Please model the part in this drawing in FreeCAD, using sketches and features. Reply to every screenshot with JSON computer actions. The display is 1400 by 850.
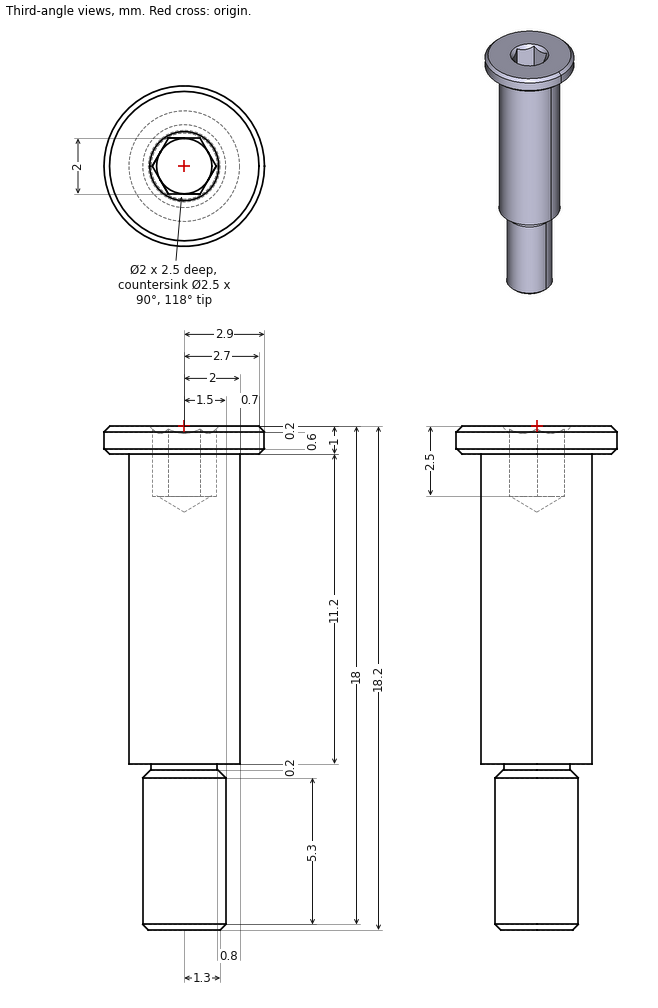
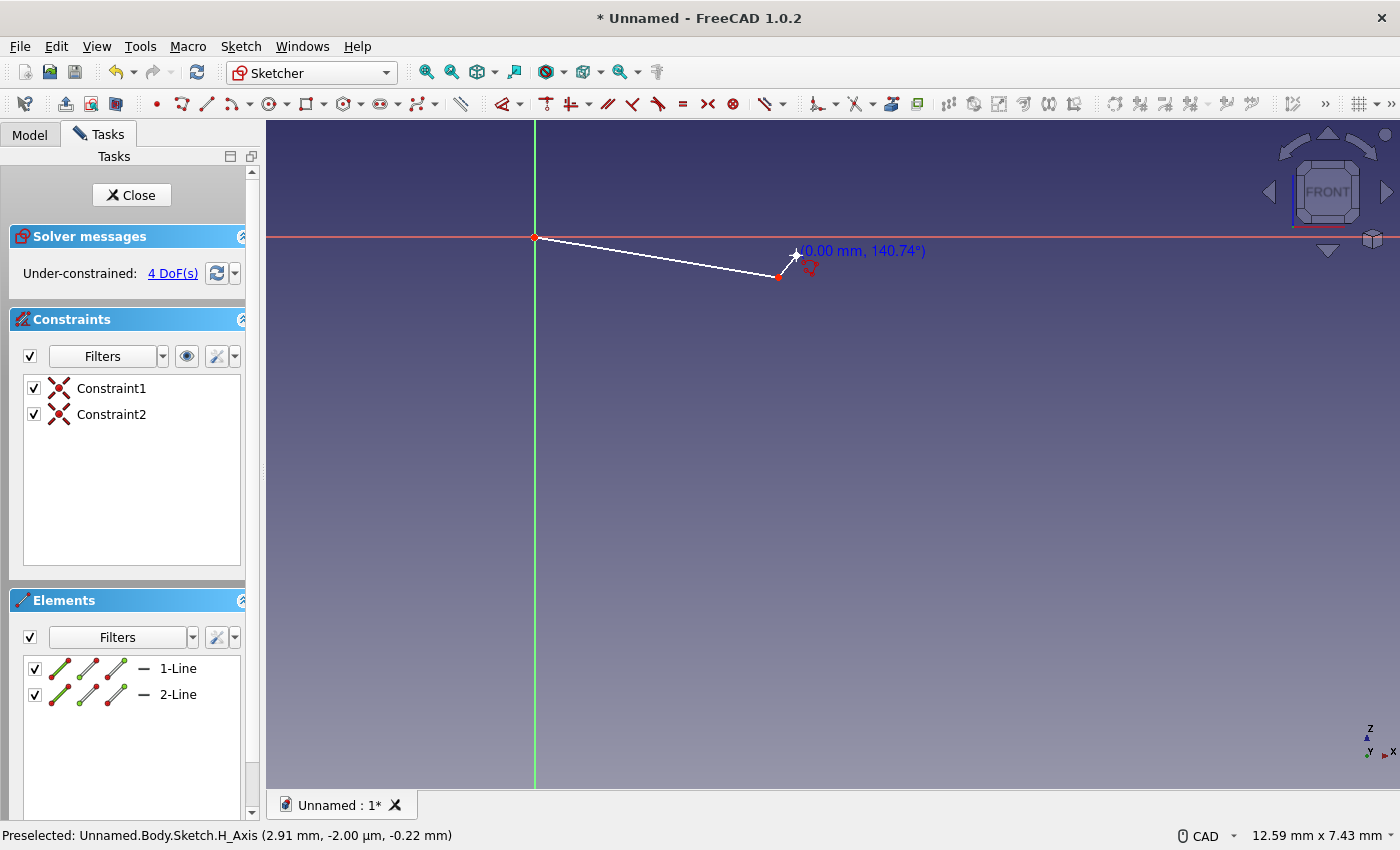
{"action": "scroll", "coordinate": [797, 257], "scroll_direction": "down", "scroll_amount": 7}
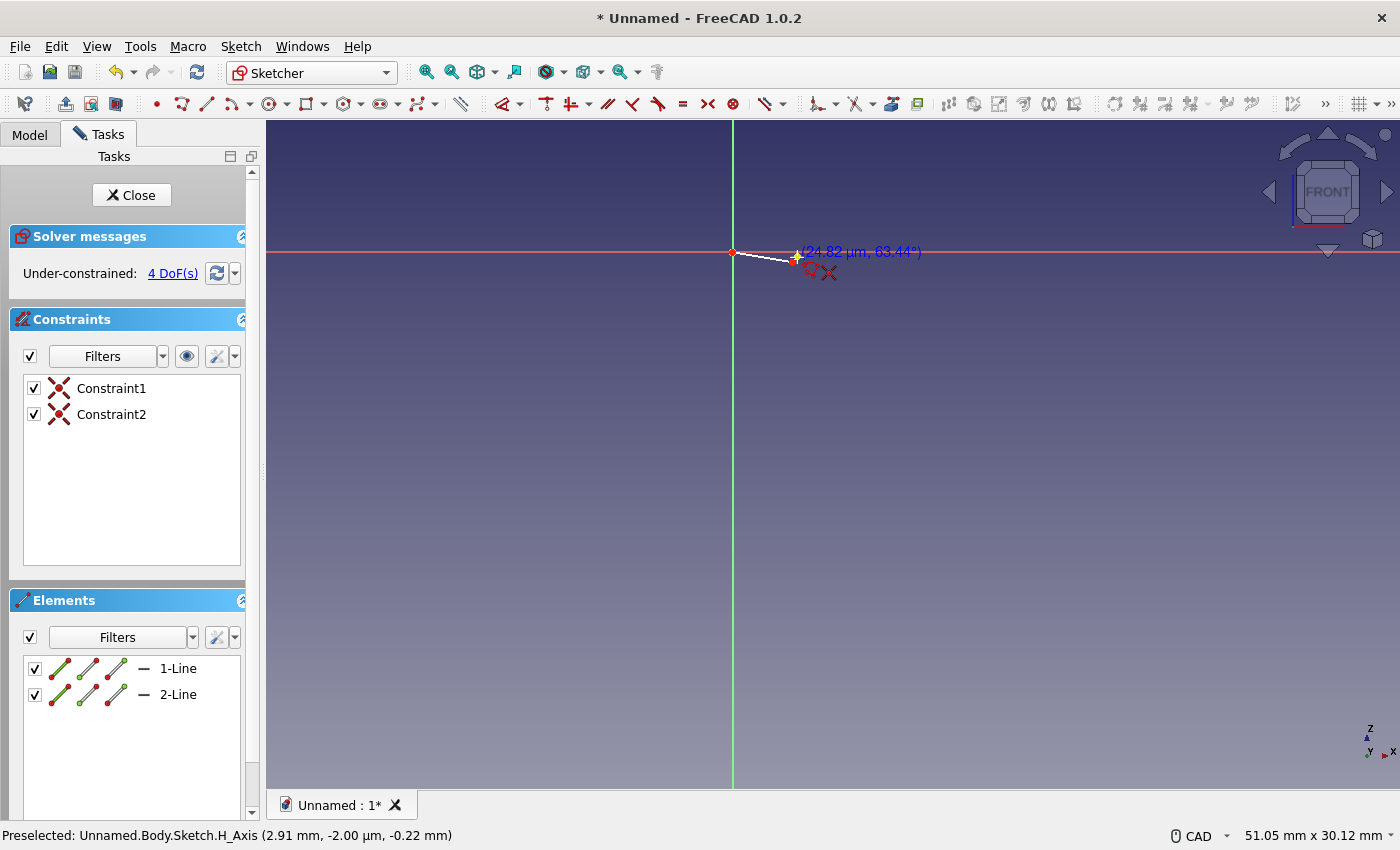
{"action": "left_click", "coordinate": [797, 270]}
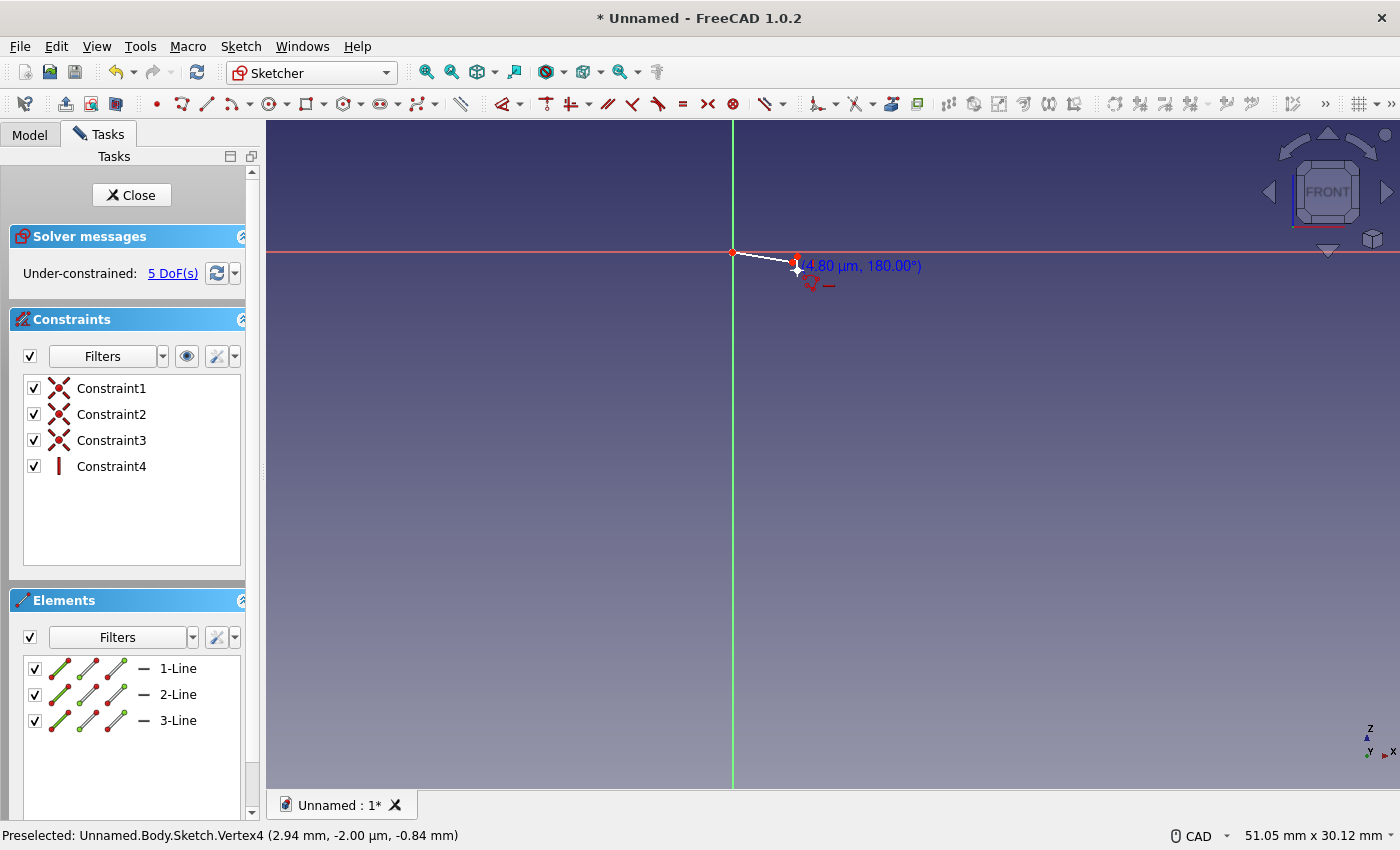
{"action": "scroll", "coordinate": [793, 274], "scroll_direction": "up", "scroll_amount": 5}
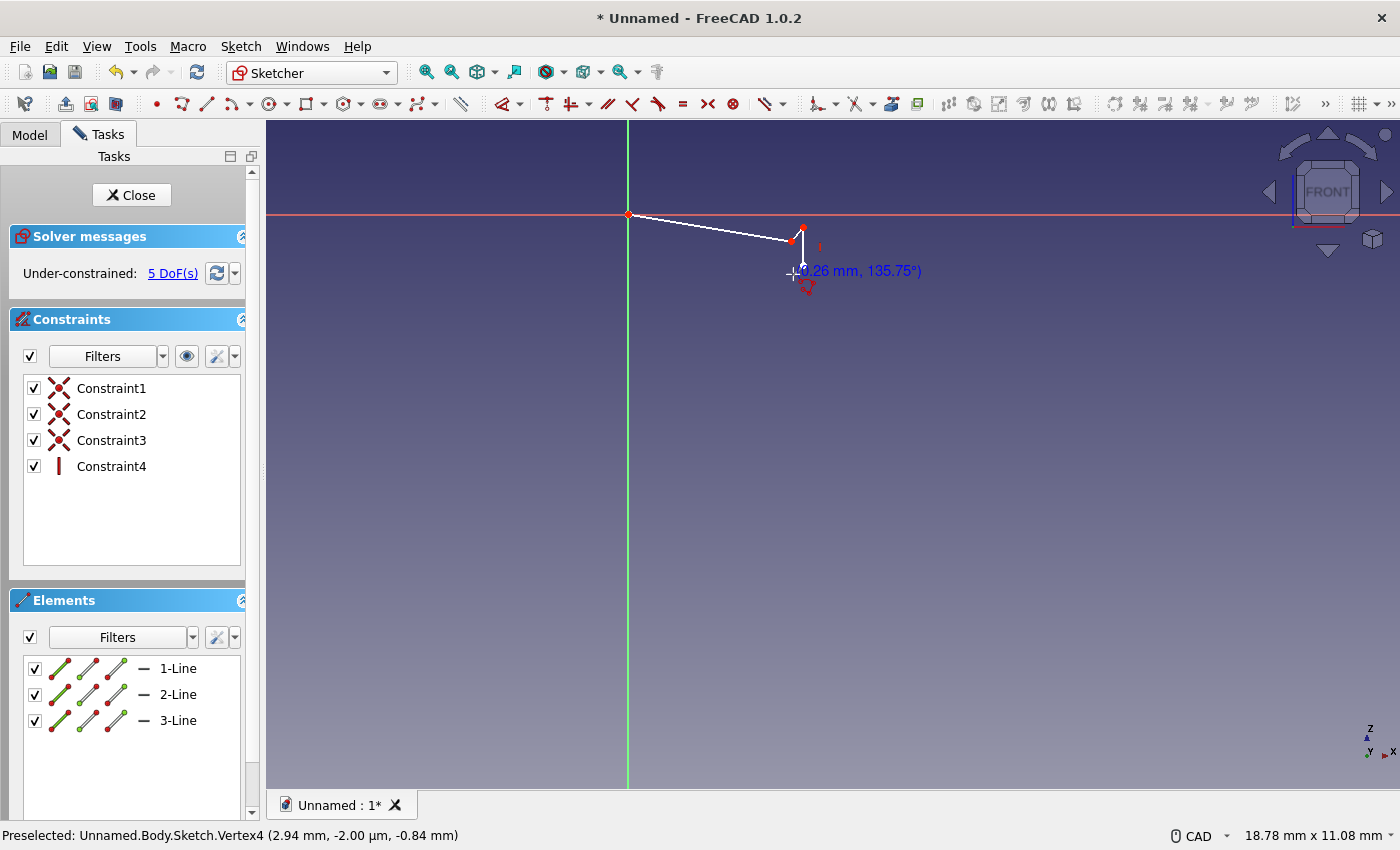
{"action": "left_click", "coordinate": [791, 275]}
{"action": "left_click", "coordinate": [749, 275]}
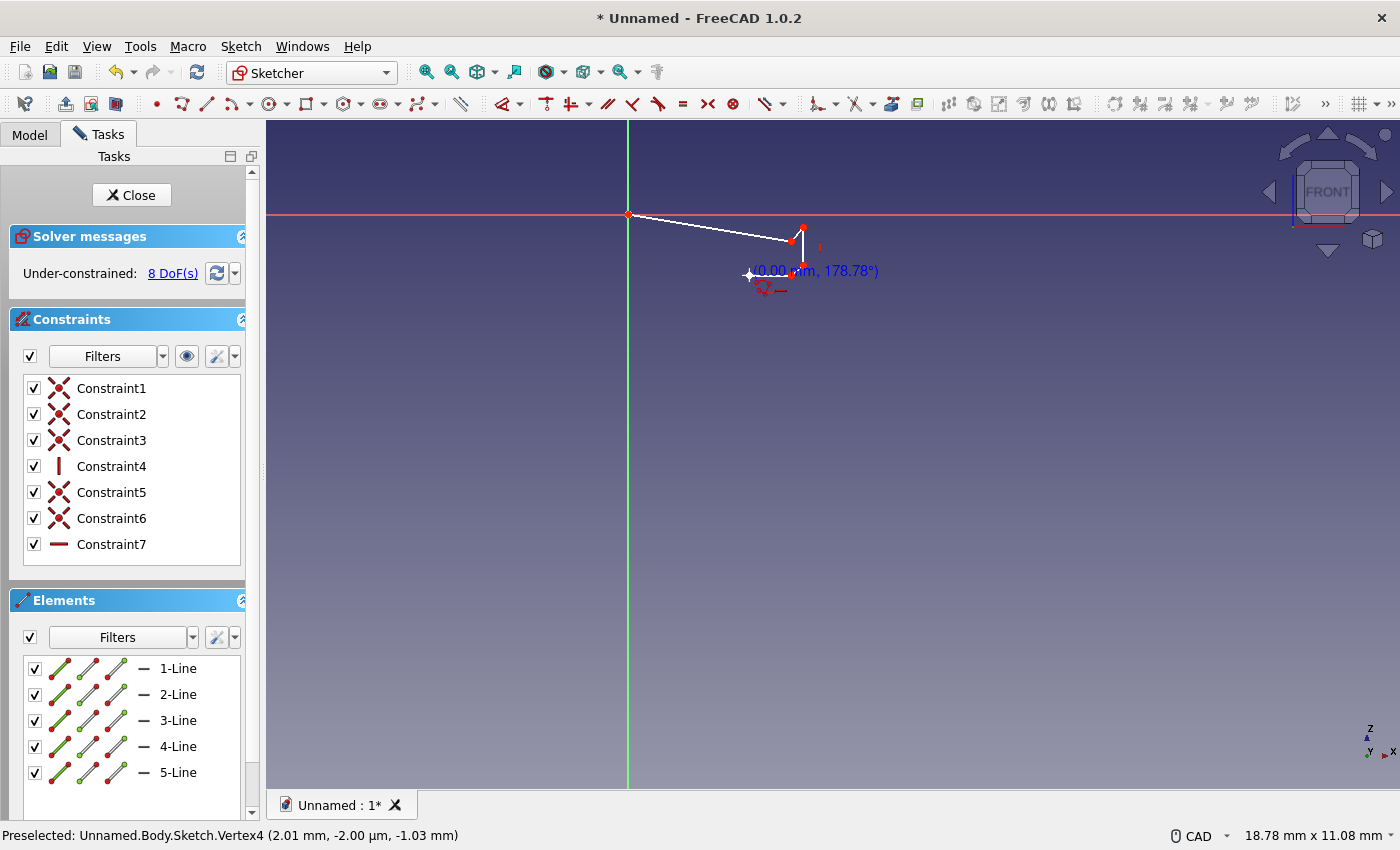
{"action": "scroll", "coordinate": [793, 274], "scroll_direction": "down", "scroll_amount": 5}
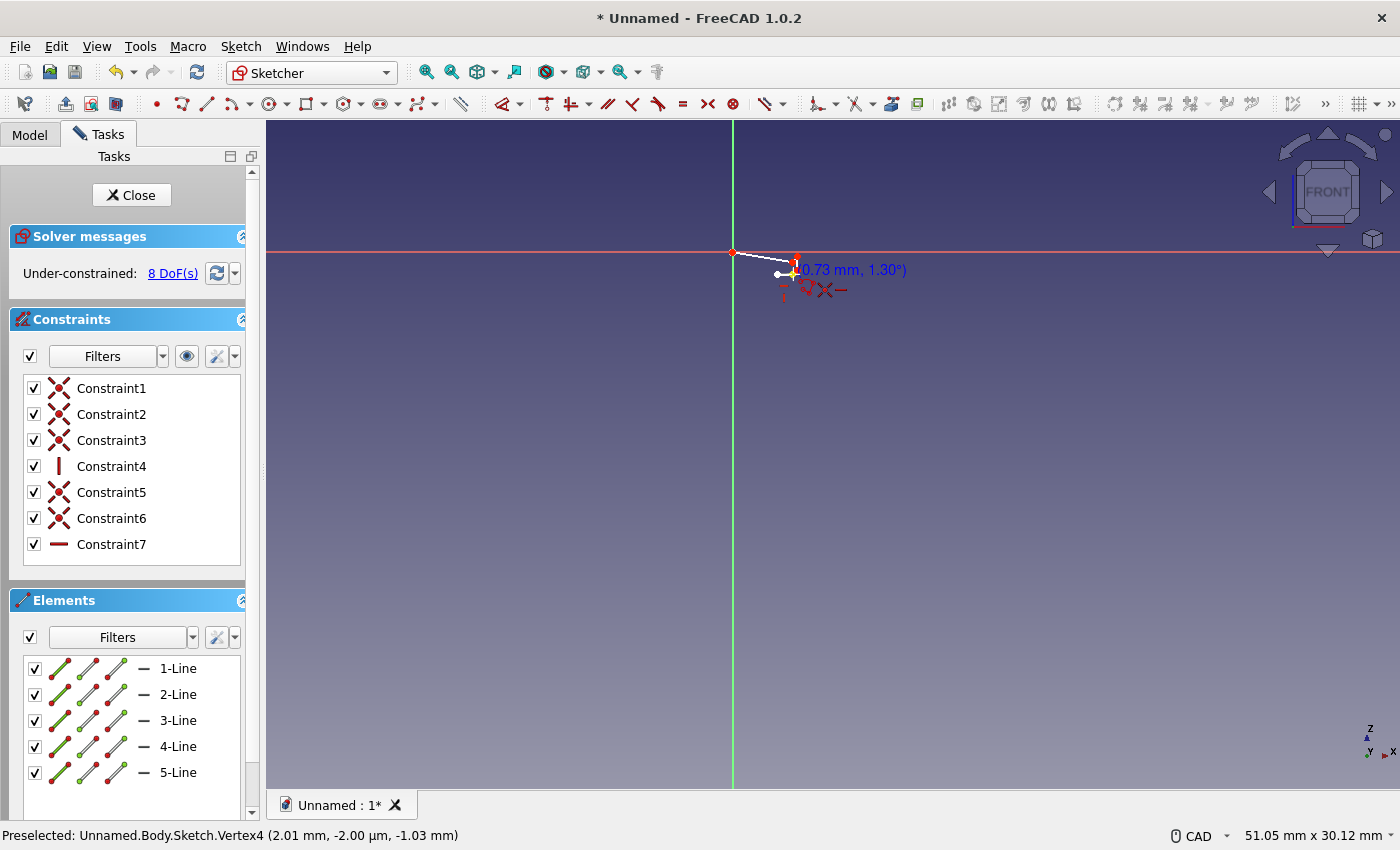
{"action": "left_click", "coordinate": [777, 523]}
{"action": "left_click", "coordinate": [759, 523]}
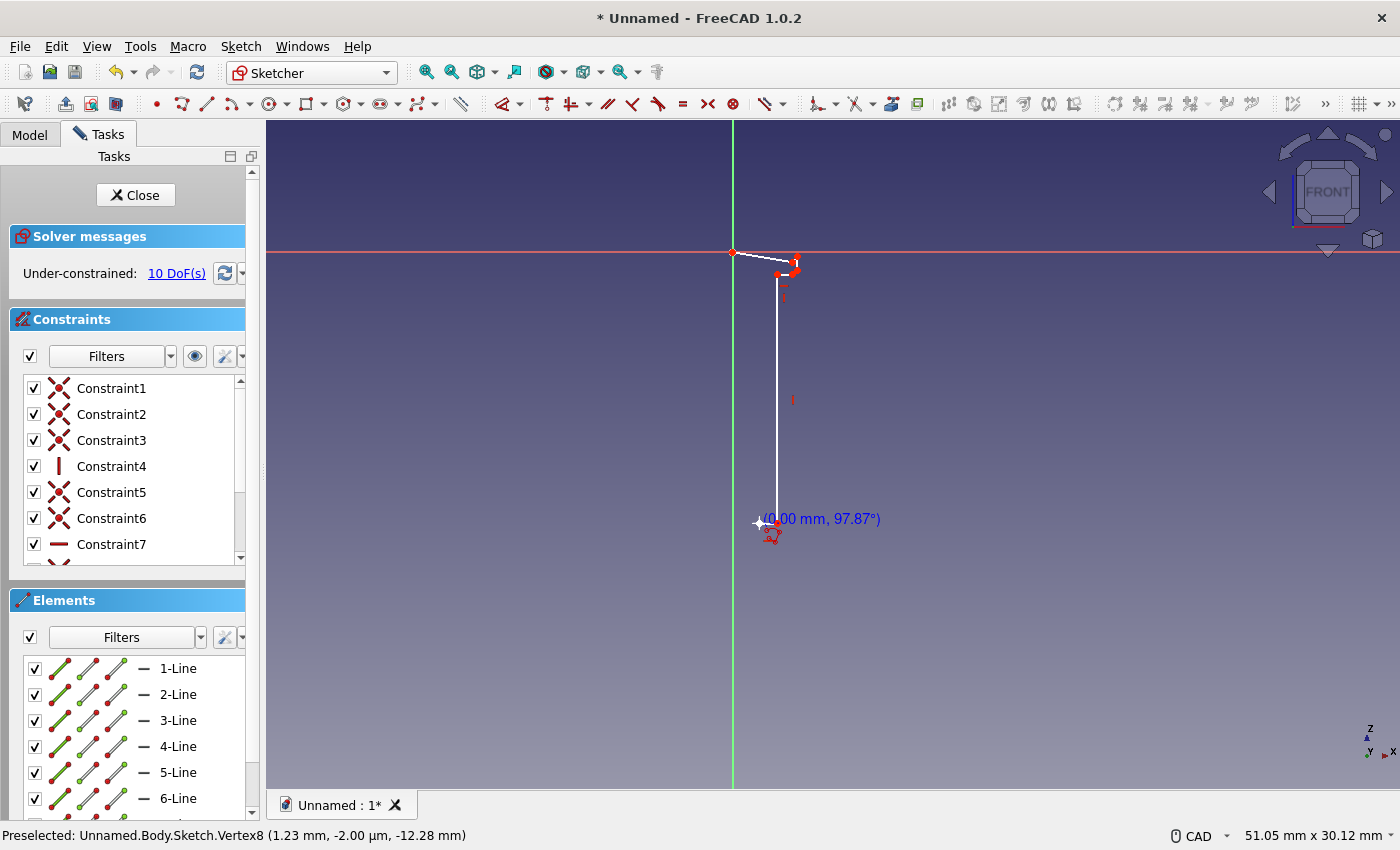
{"action": "scroll", "coordinate": [759, 528], "scroll_direction": "up", "scroll_amount": 7}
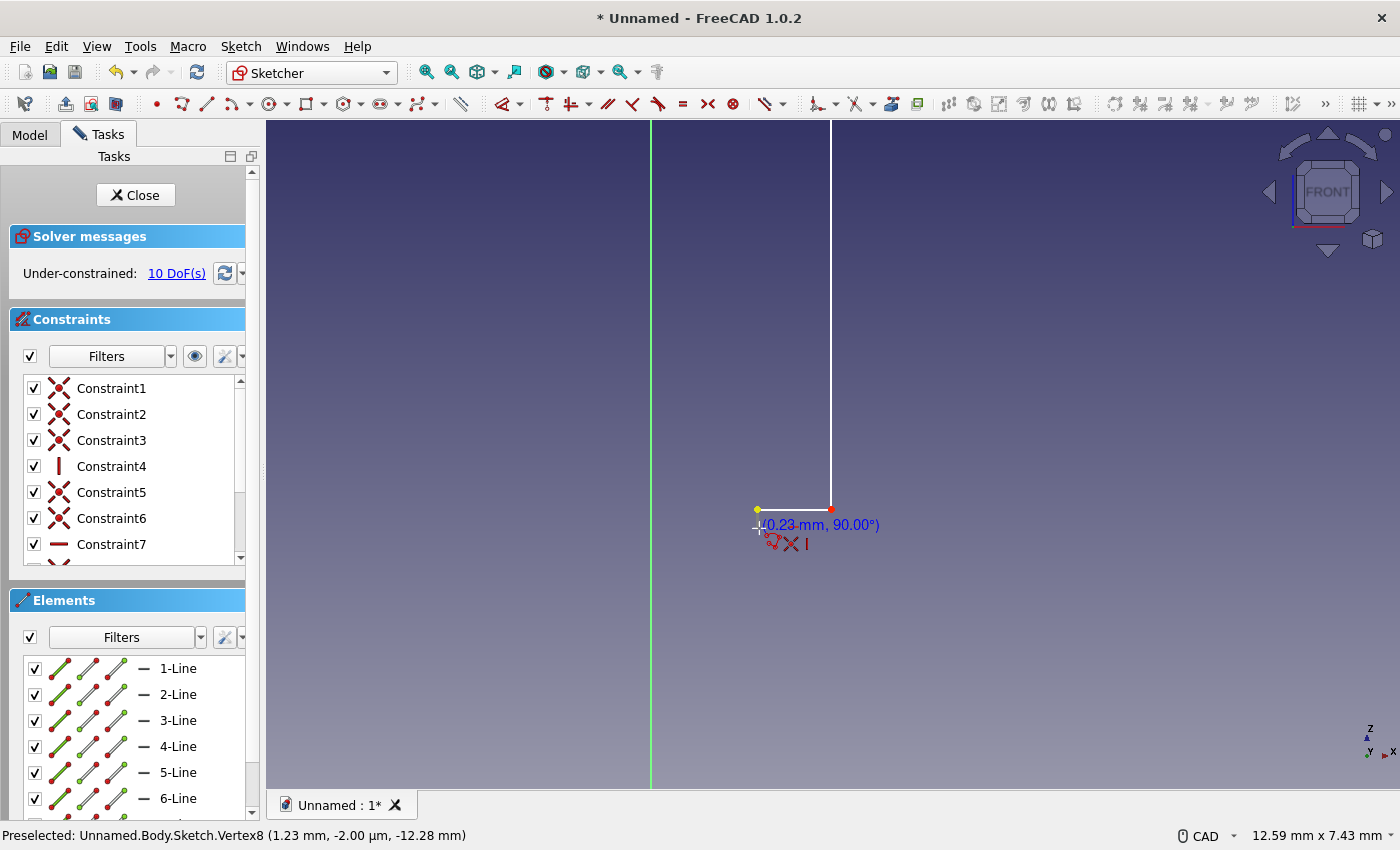
{"action": "left_click", "coordinate": [758, 525]}
{"action": "left_click", "coordinate": [786, 552]}